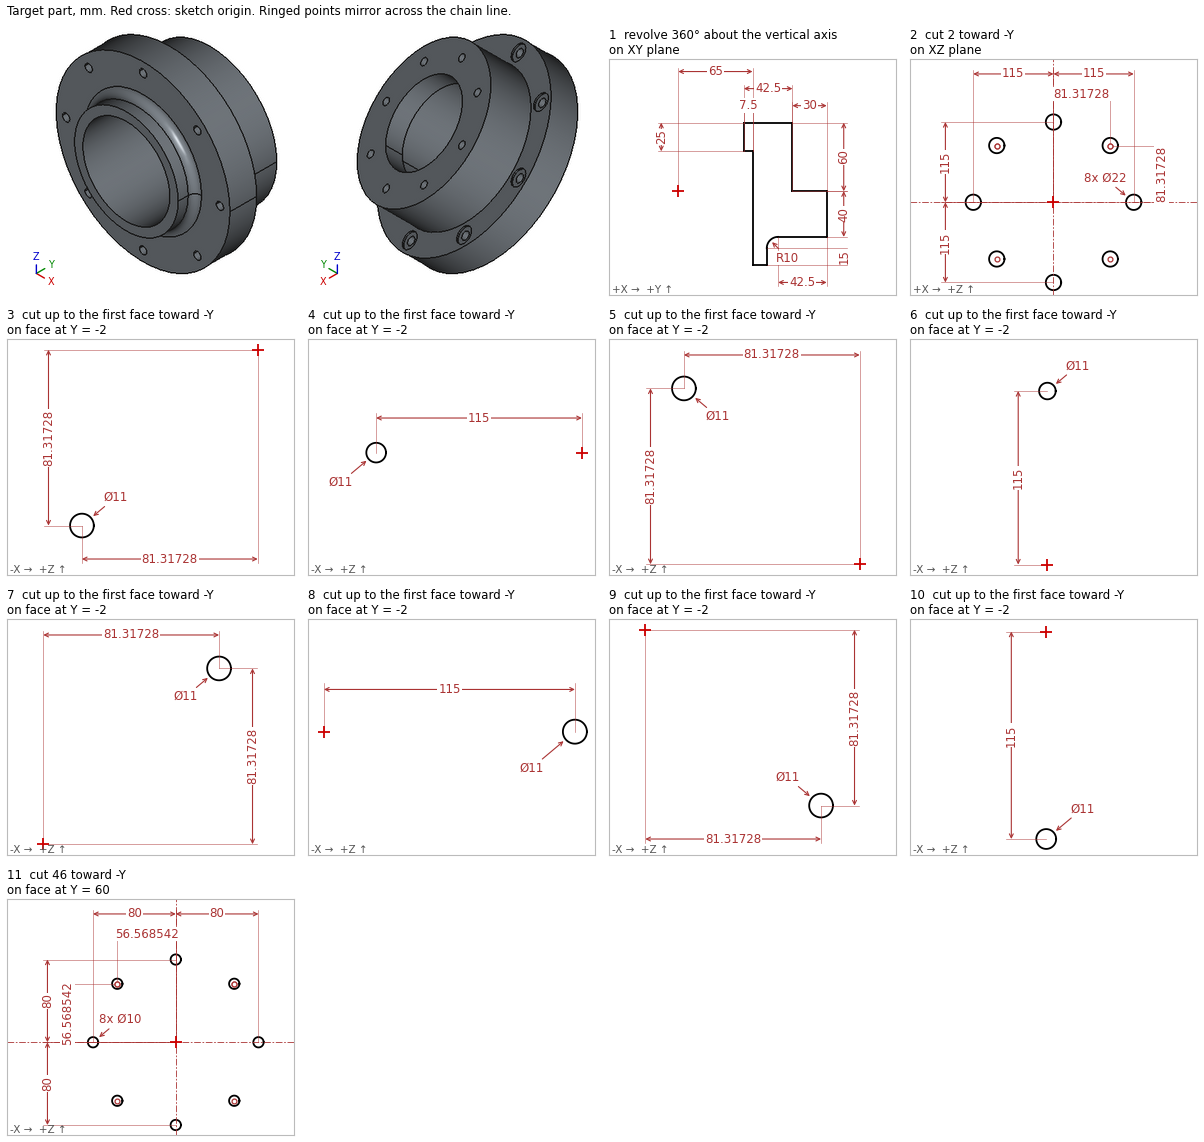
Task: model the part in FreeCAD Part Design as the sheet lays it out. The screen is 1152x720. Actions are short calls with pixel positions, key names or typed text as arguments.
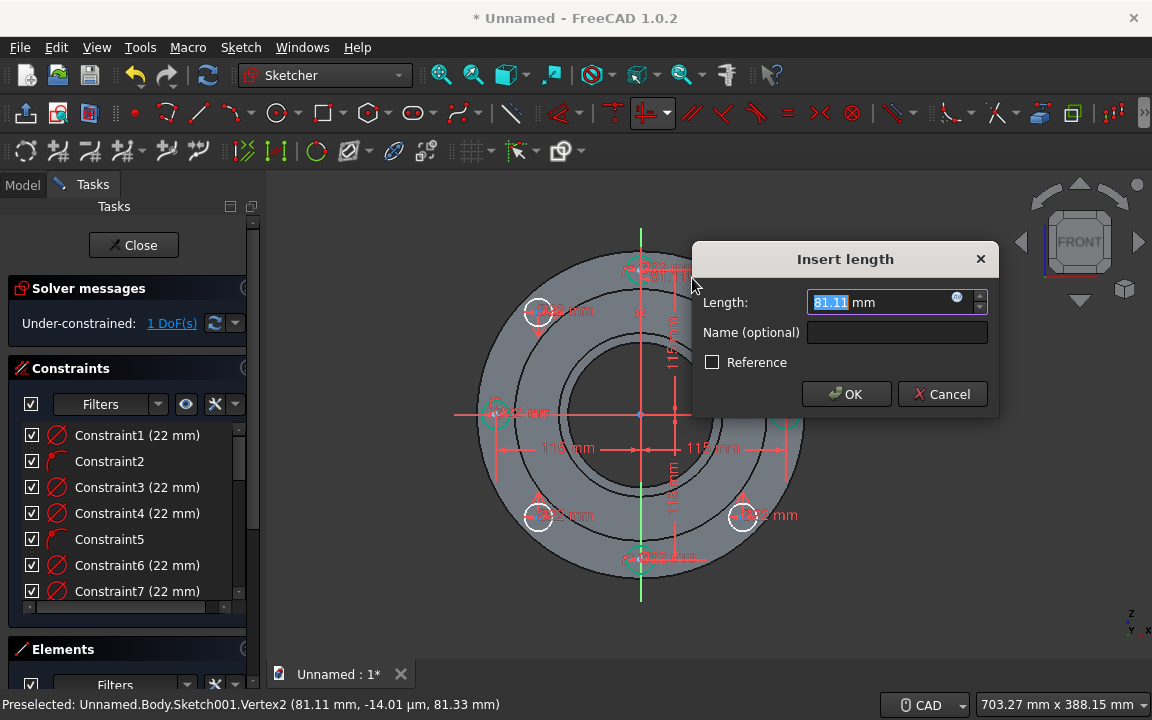
text(81.31728)
key(Return)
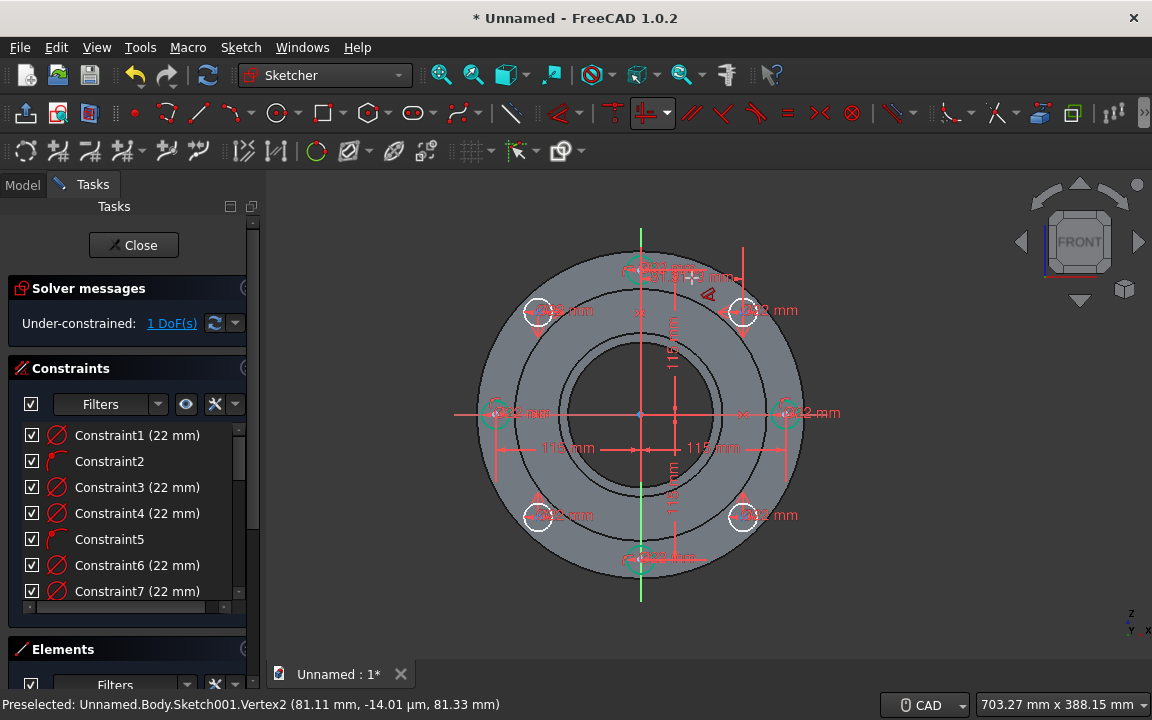
click(743, 312)
click(777, 364)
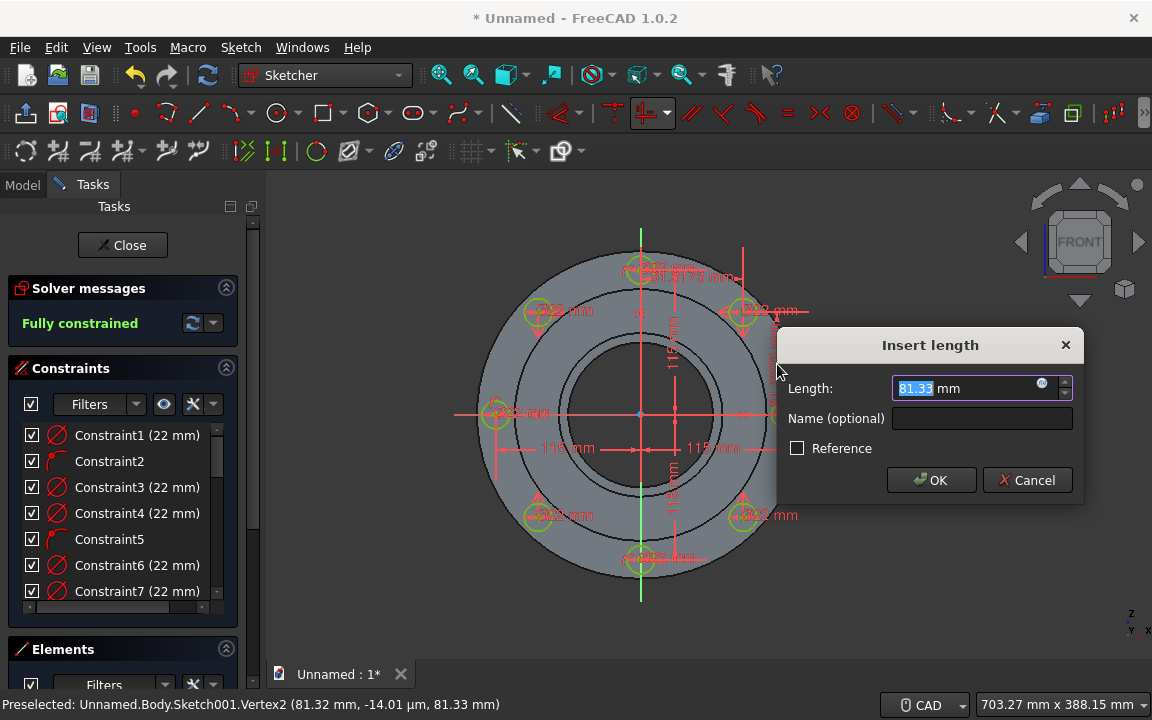
text(81.31728)
key(Return)
key(Escape)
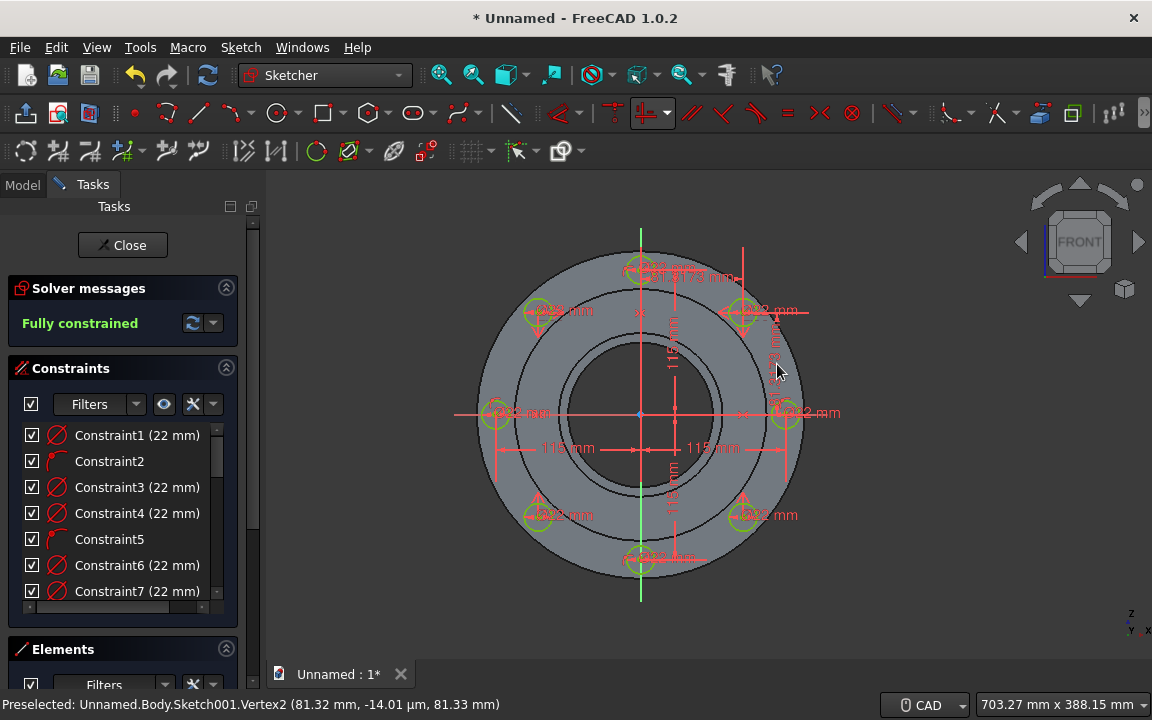
click(123, 245)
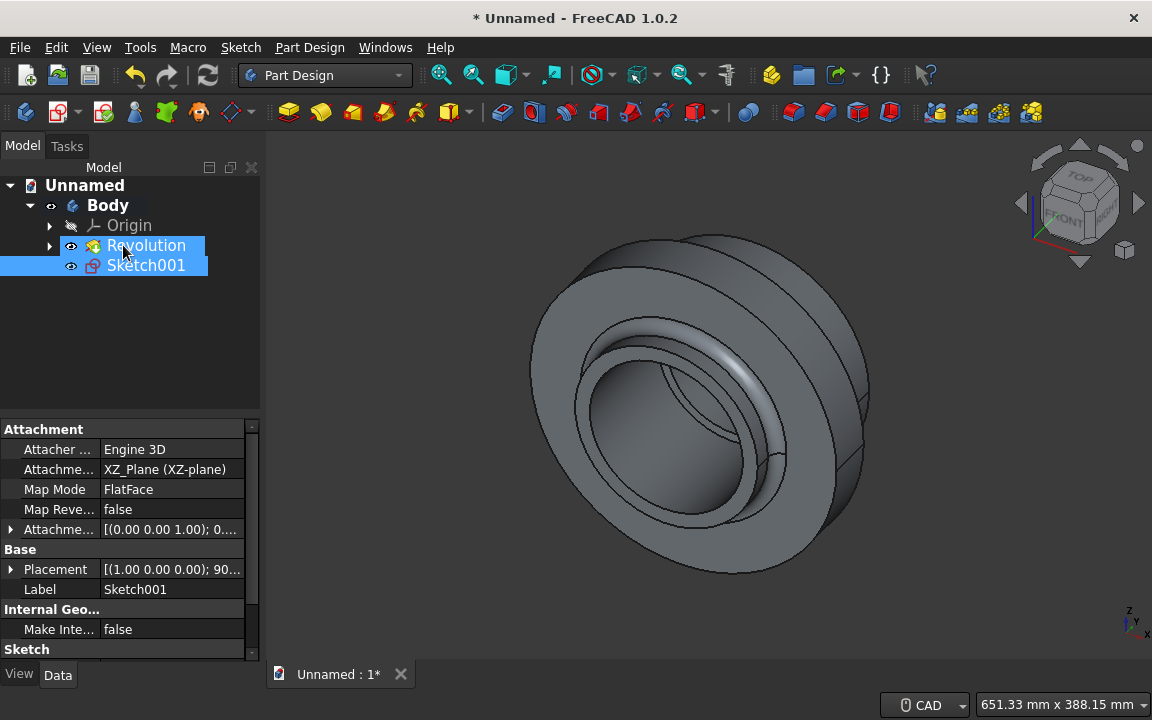
click(504, 112)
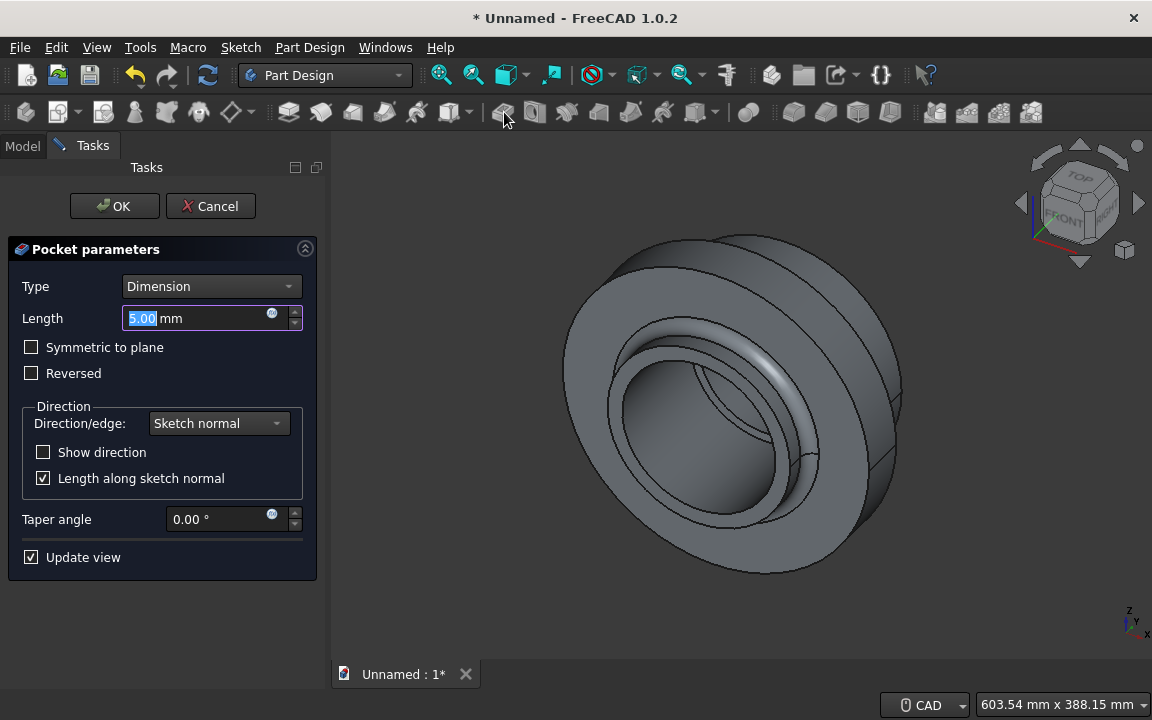
text(2)
key(Tab)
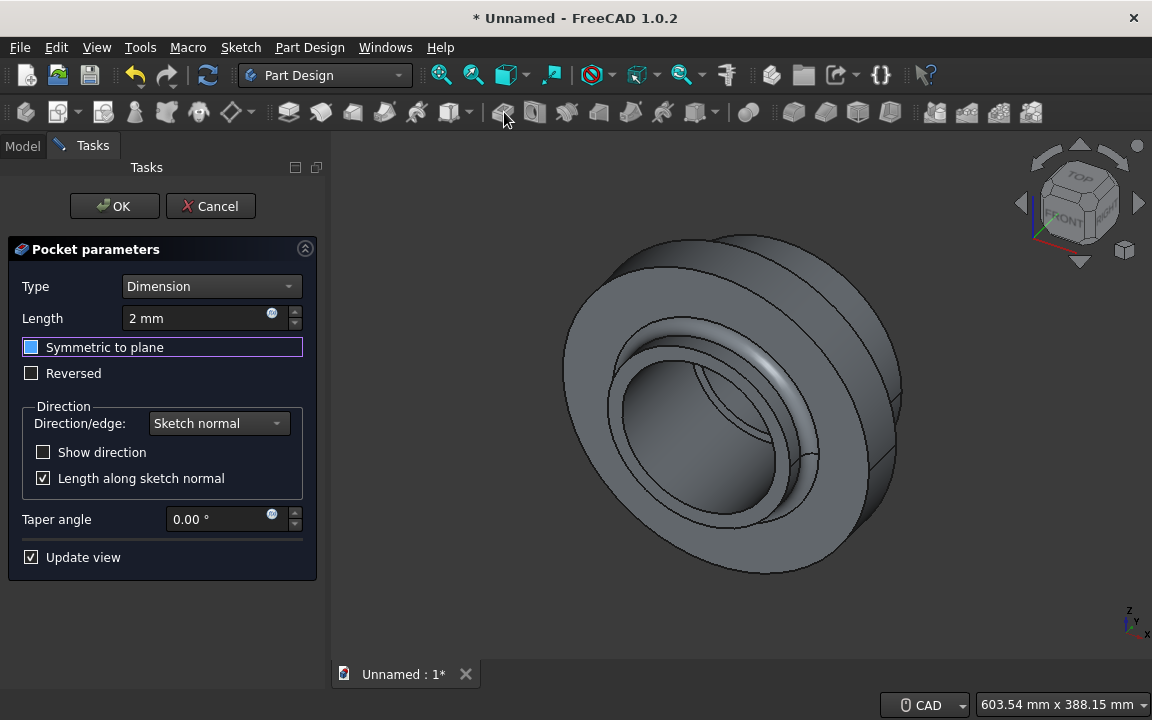
click(30, 373)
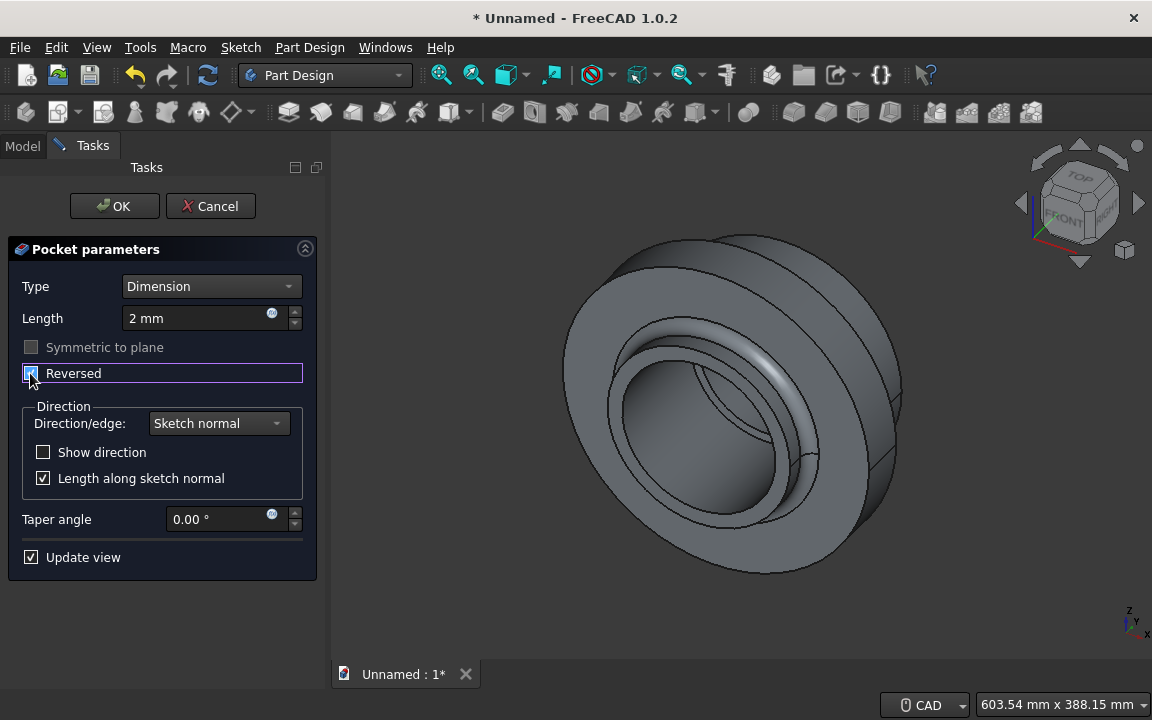
click(115, 206)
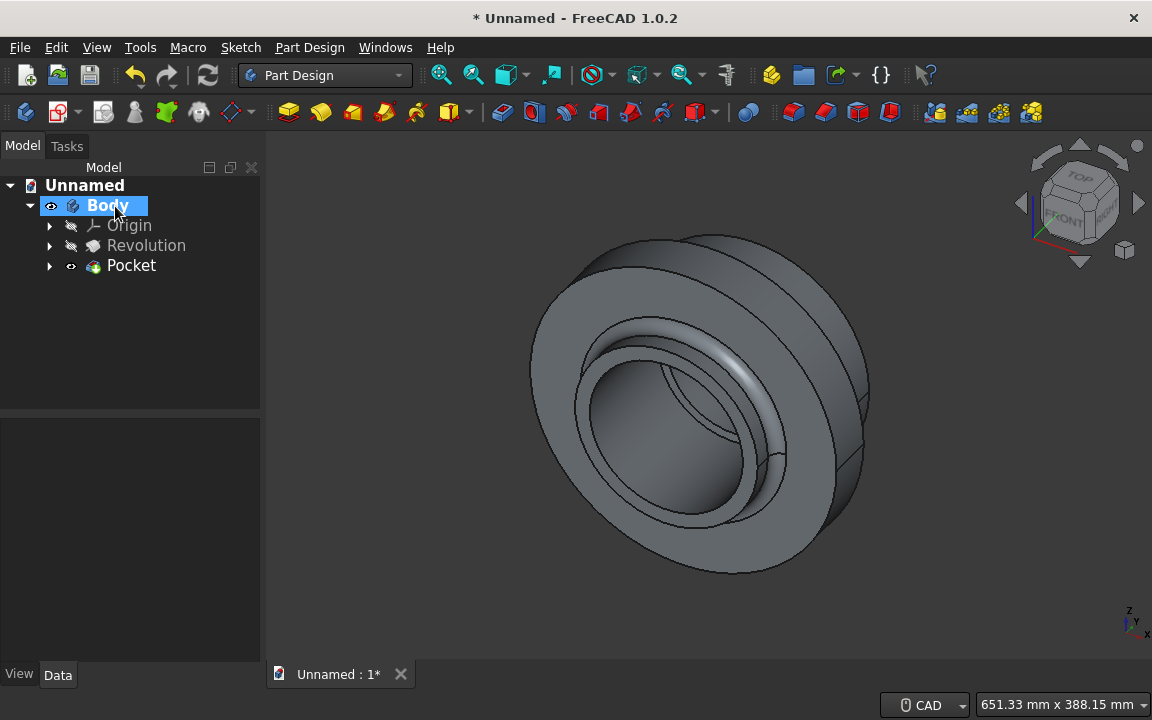
key(4)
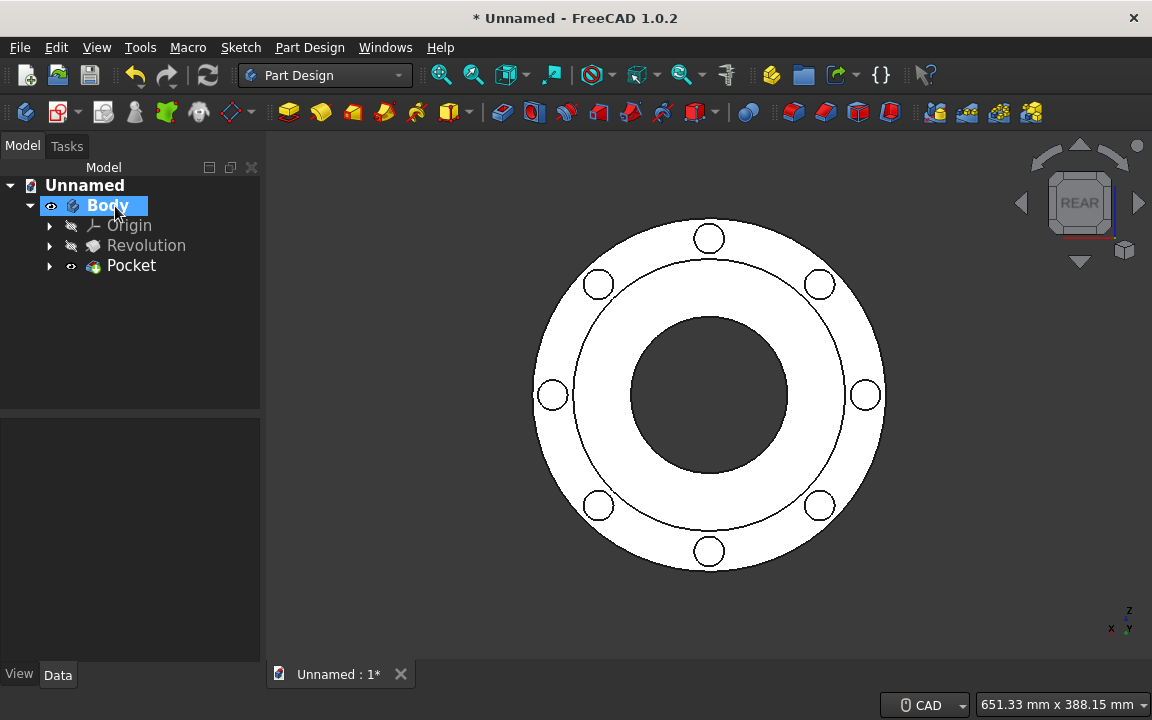
click(599, 283)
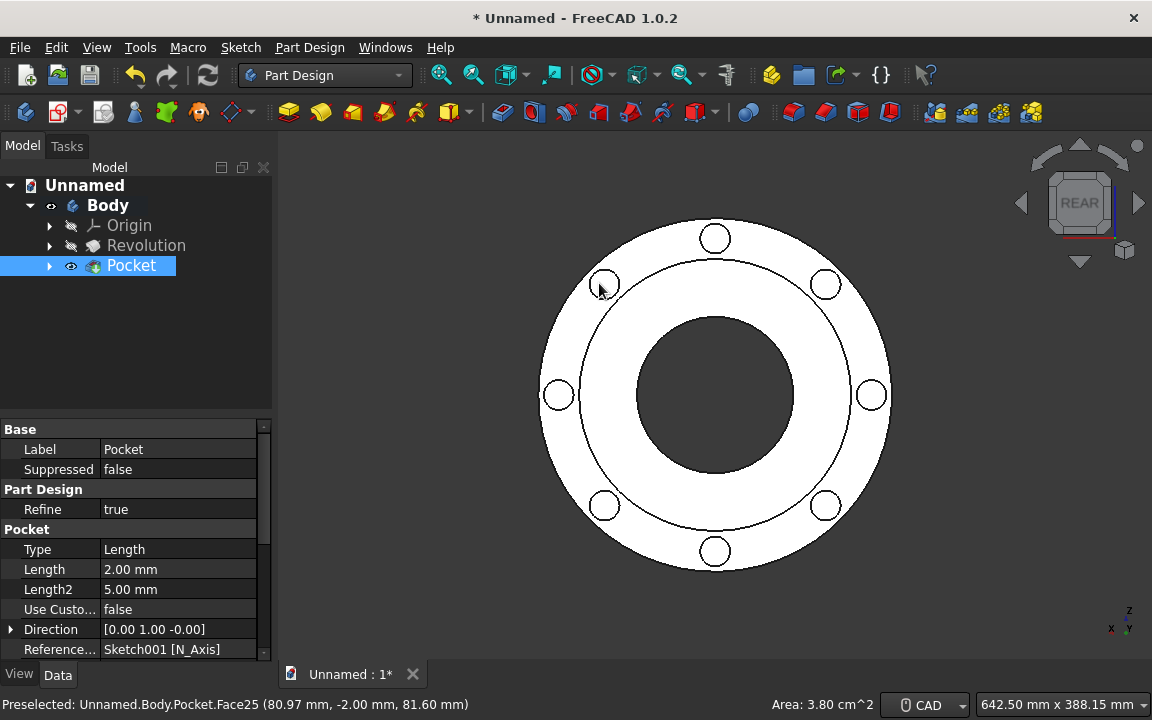
click(58, 112)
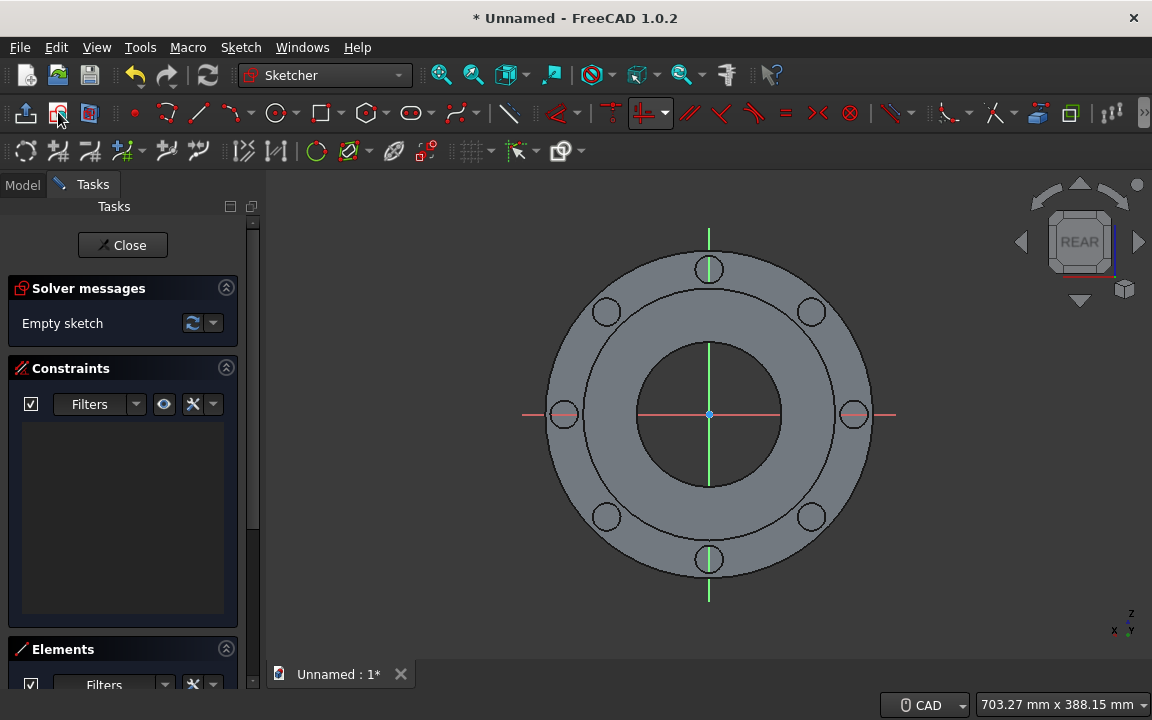
scroll(605, 522, up, 15)